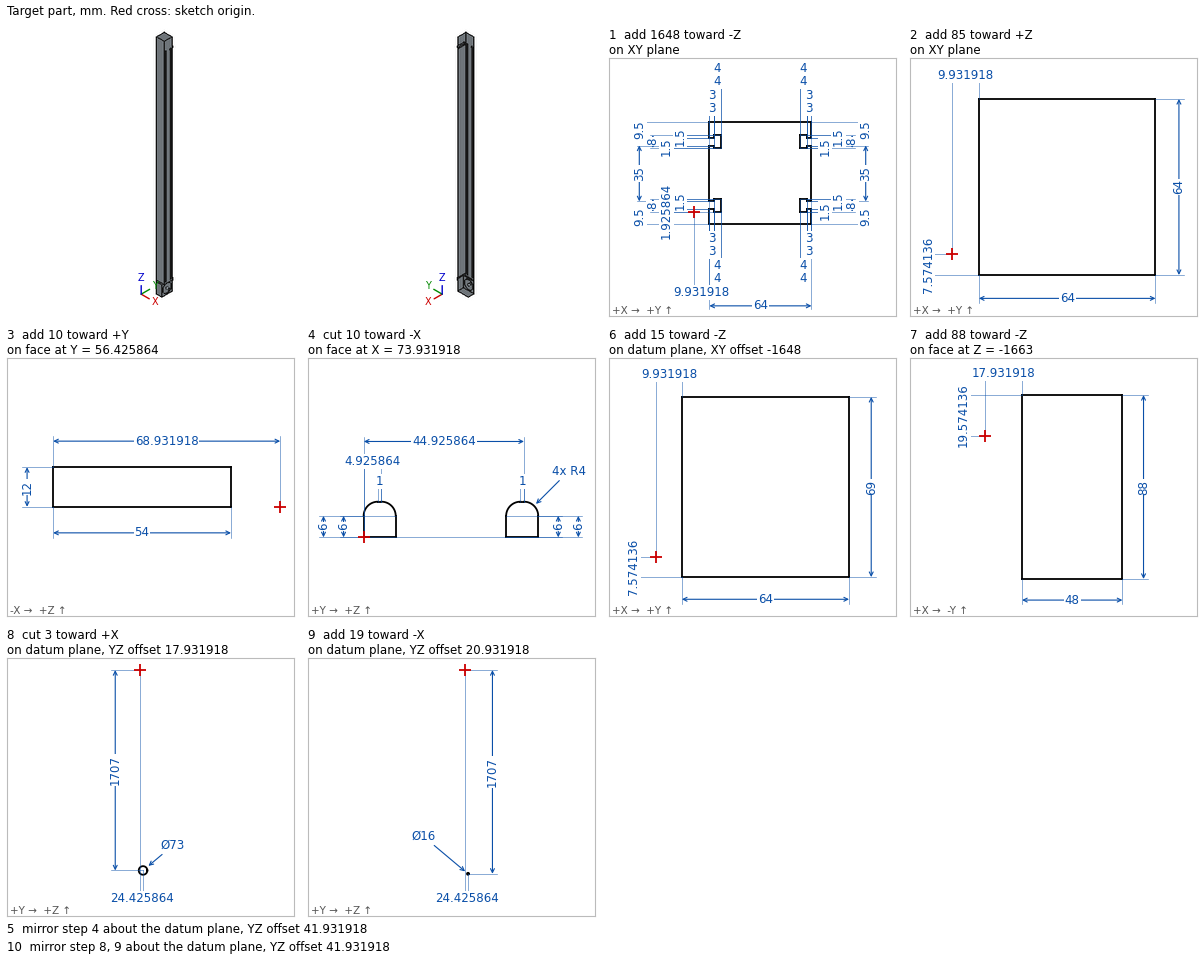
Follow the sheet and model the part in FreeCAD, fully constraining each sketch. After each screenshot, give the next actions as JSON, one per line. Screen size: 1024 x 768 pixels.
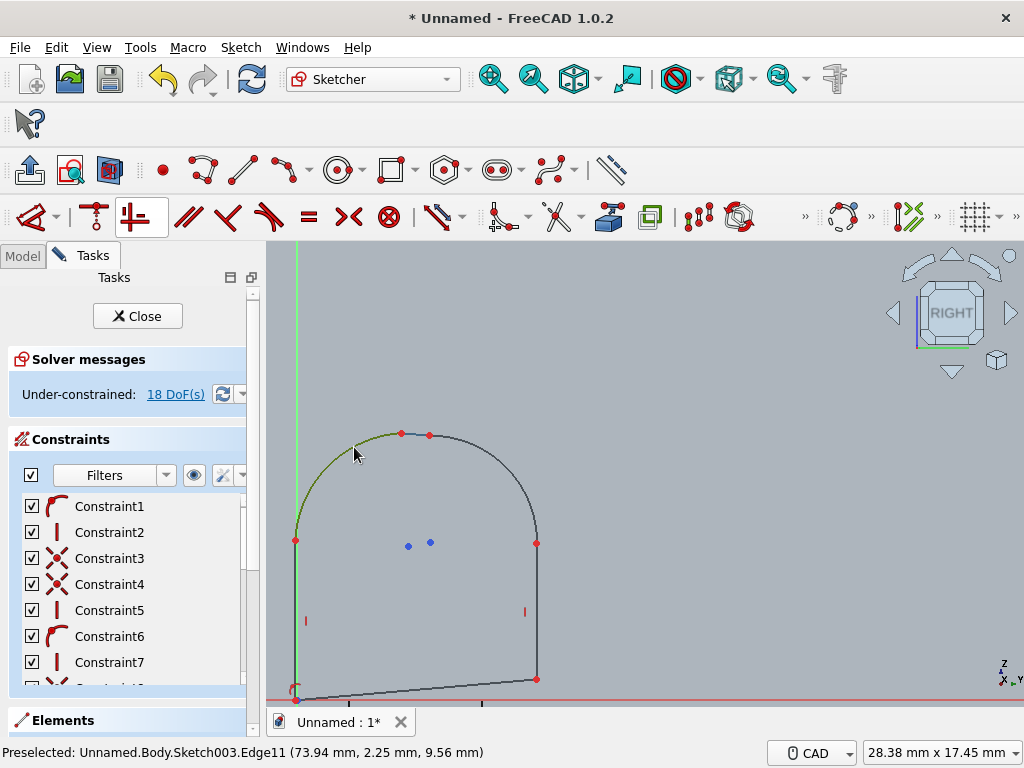
{"action": "left_click", "coordinate": [270, 218]}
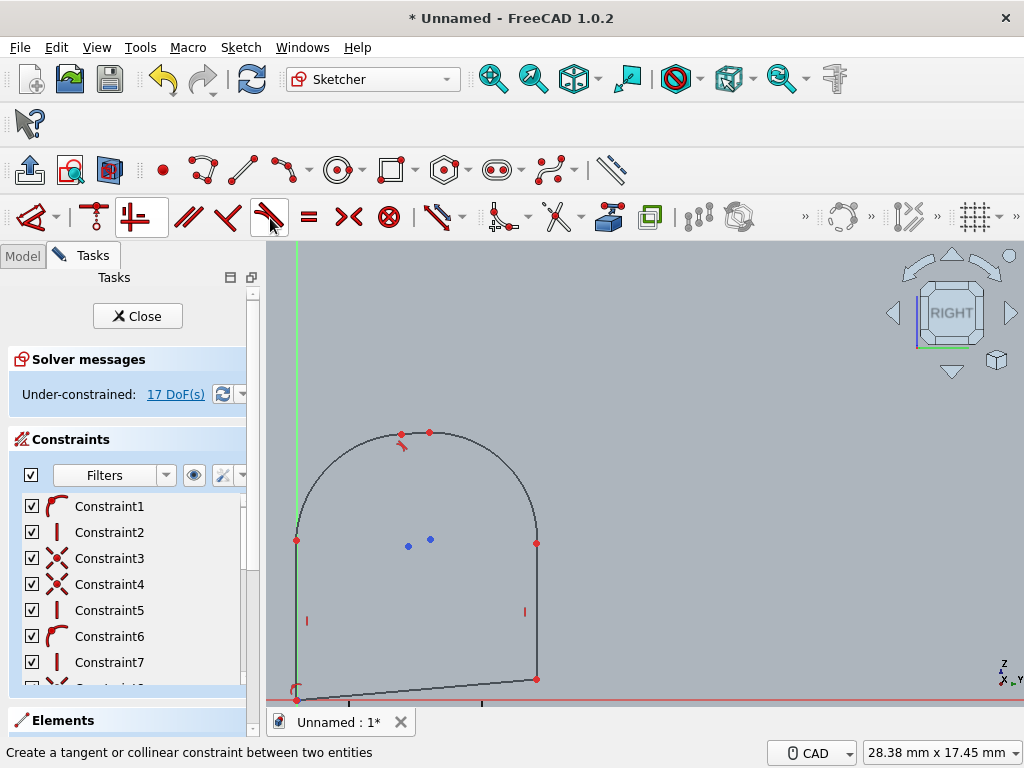
{"action": "scroll", "coordinate": [418, 433], "scroll_direction": "up", "scroll_amount": 2}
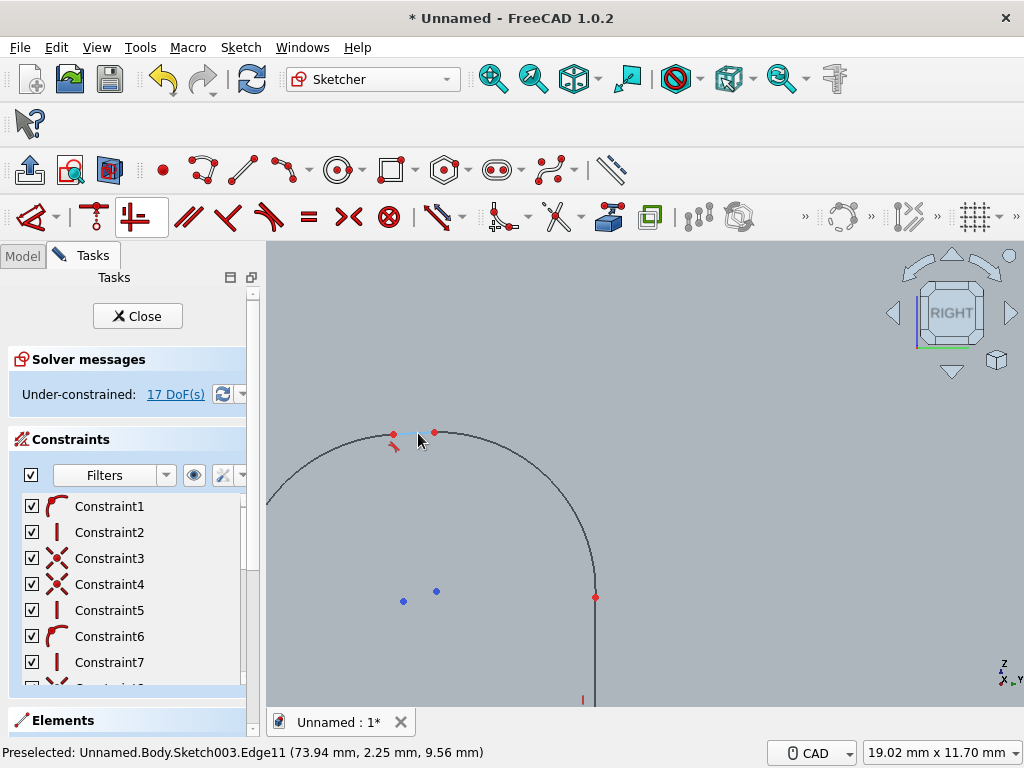
{"action": "left_click", "coordinate": [418, 433]}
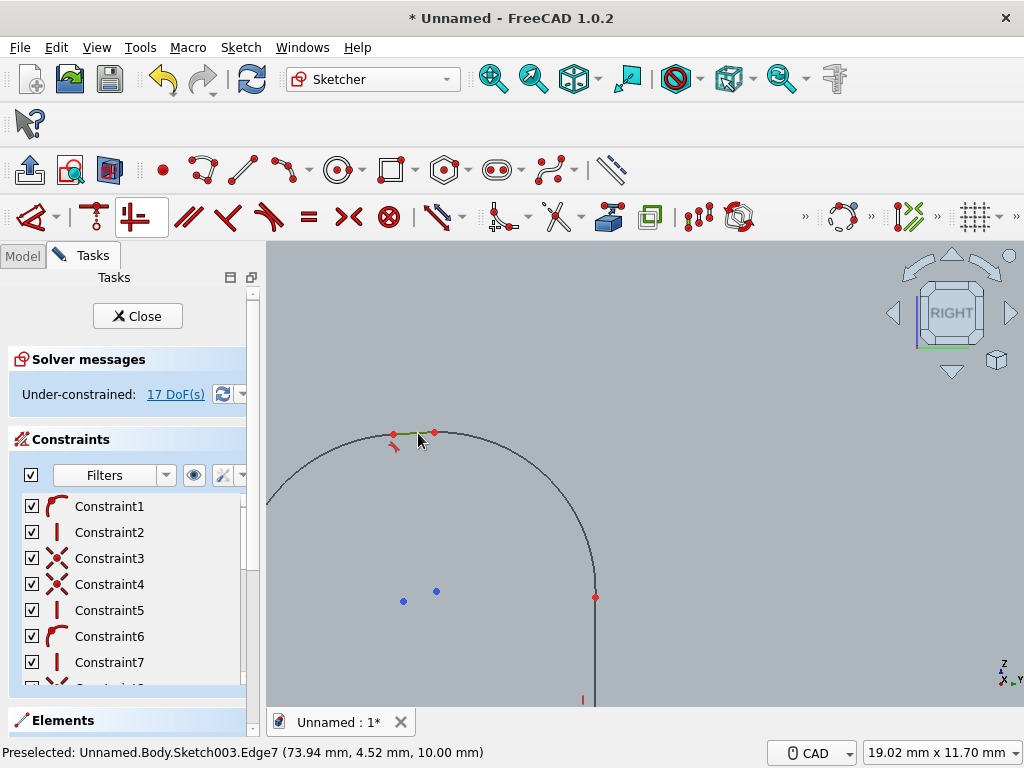
{"action": "scroll", "coordinate": [416, 434], "scroll_direction": "down", "scroll_amount": 8}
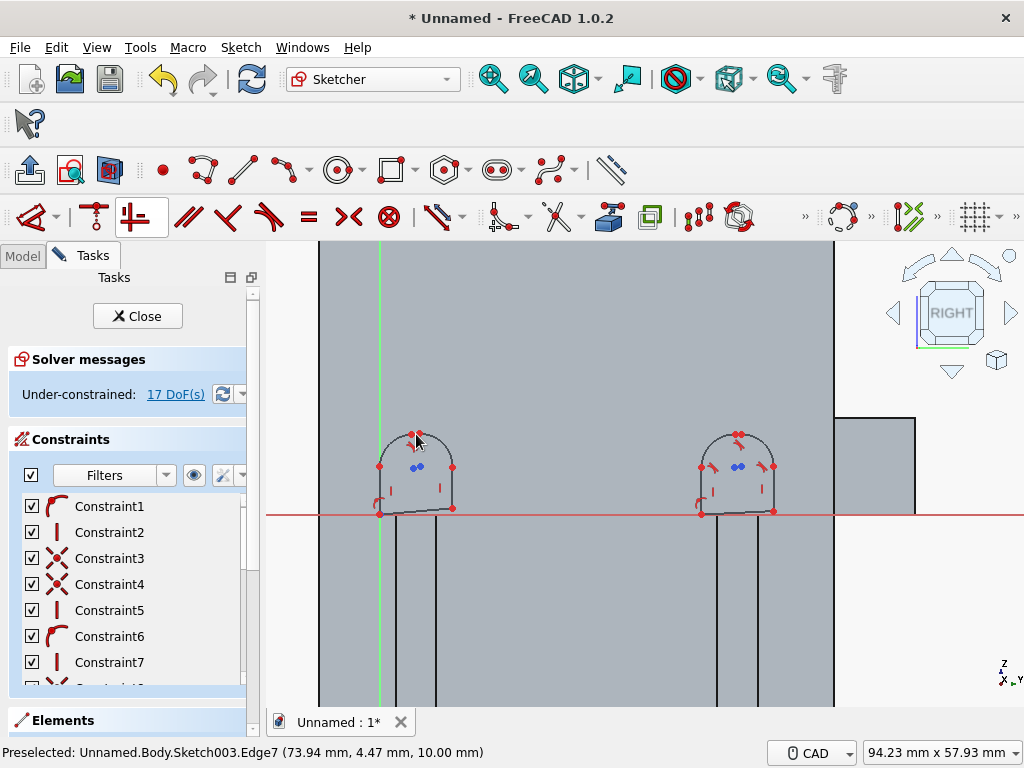
{"action": "left_click", "coordinate": [449, 452]}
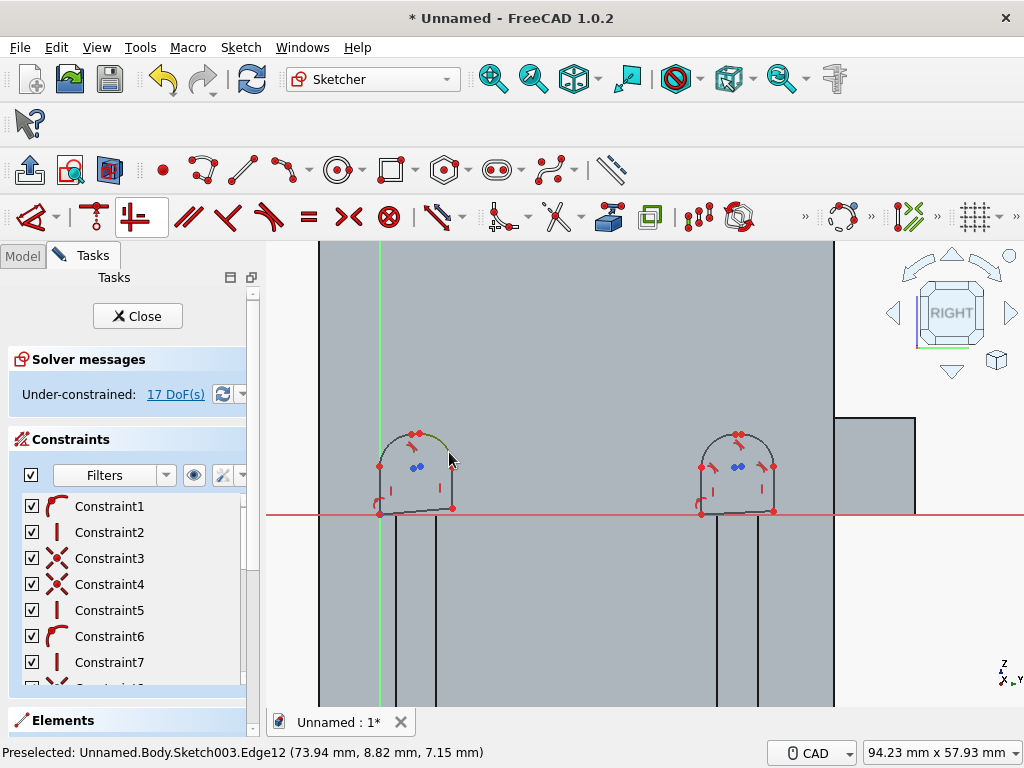
{"action": "left_click", "coordinate": [270, 218]}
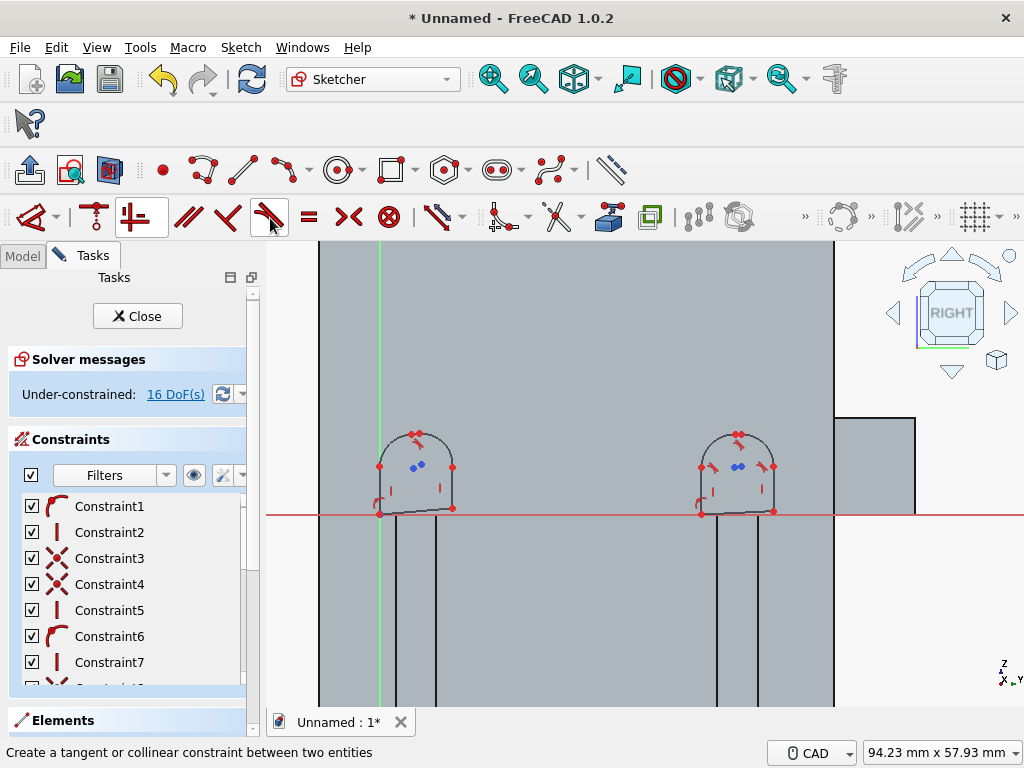
{"action": "left_click", "coordinate": [380, 481]}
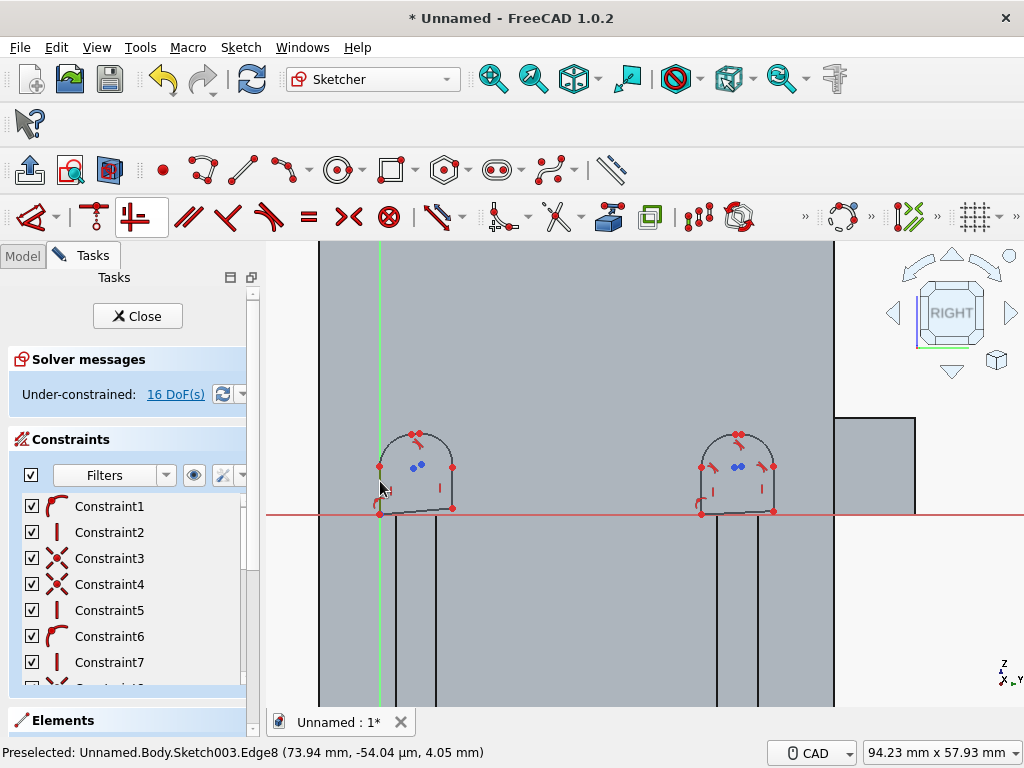
{"action": "left_click", "coordinate": [397, 438]}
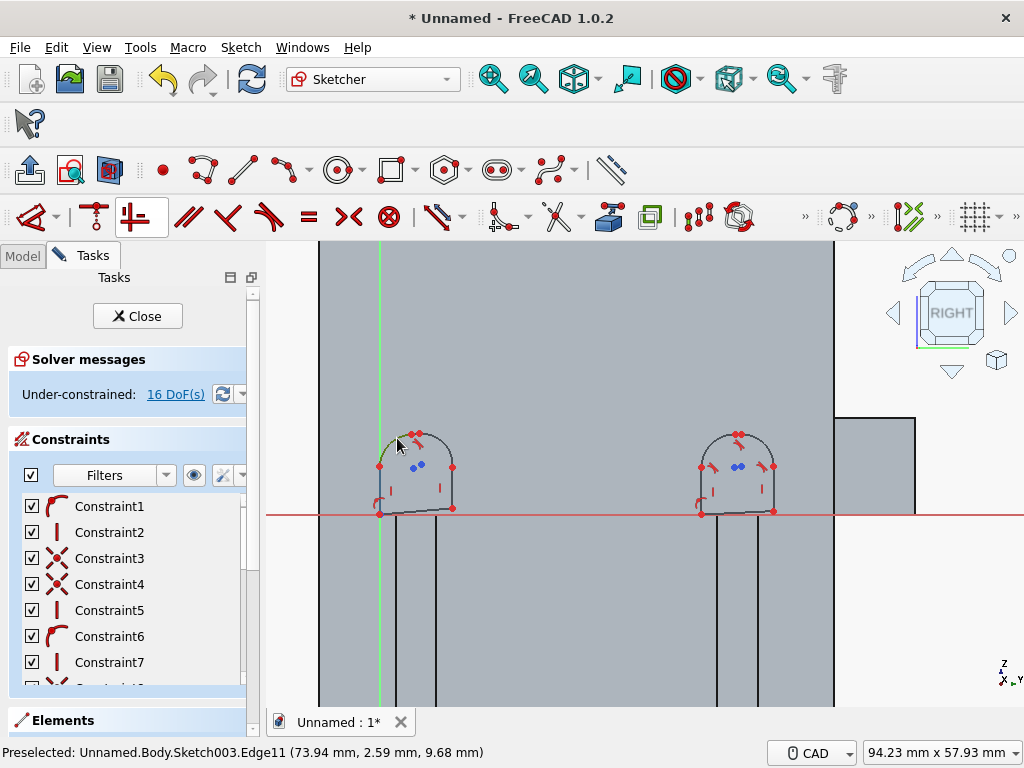
{"action": "left_click", "coordinate": [270, 218]}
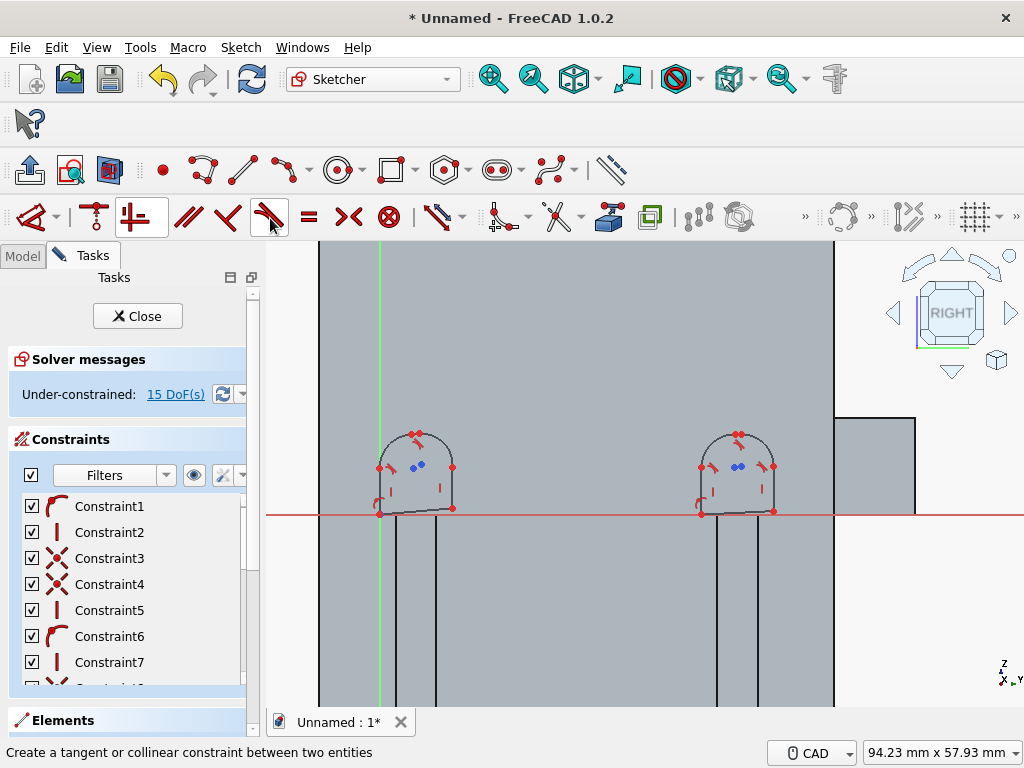
{"action": "left_click", "coordinate": [452, 496]}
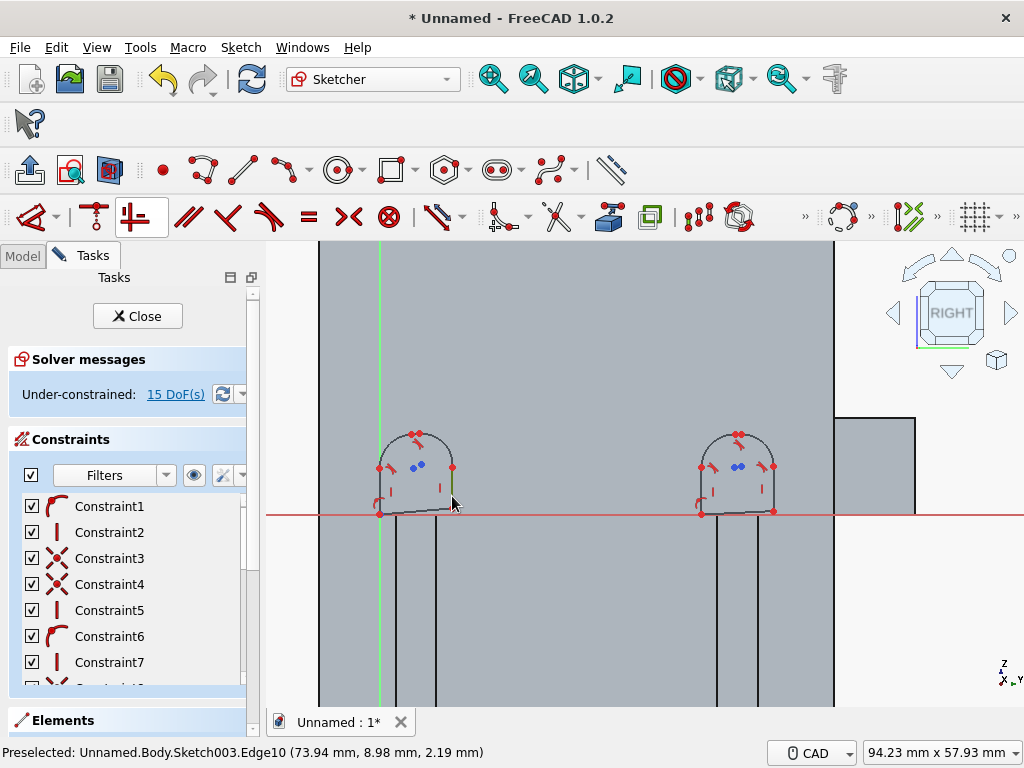
{"action": "left_click", "coordinate": [450, 452]}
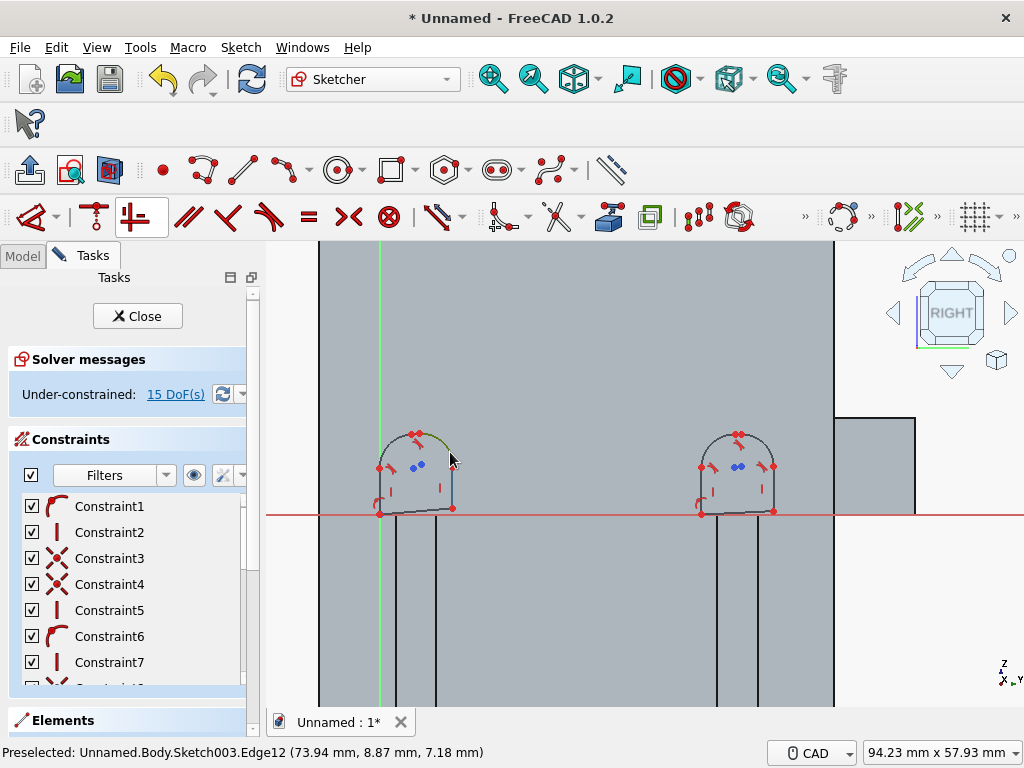
{"action": "left_click", "coordinate": [270, 218]}